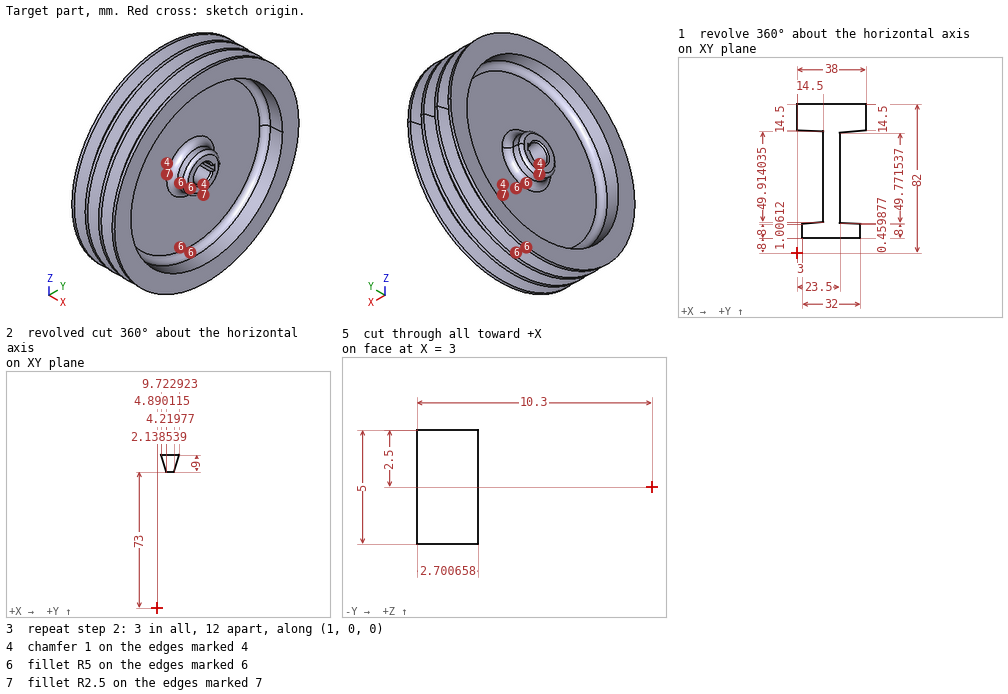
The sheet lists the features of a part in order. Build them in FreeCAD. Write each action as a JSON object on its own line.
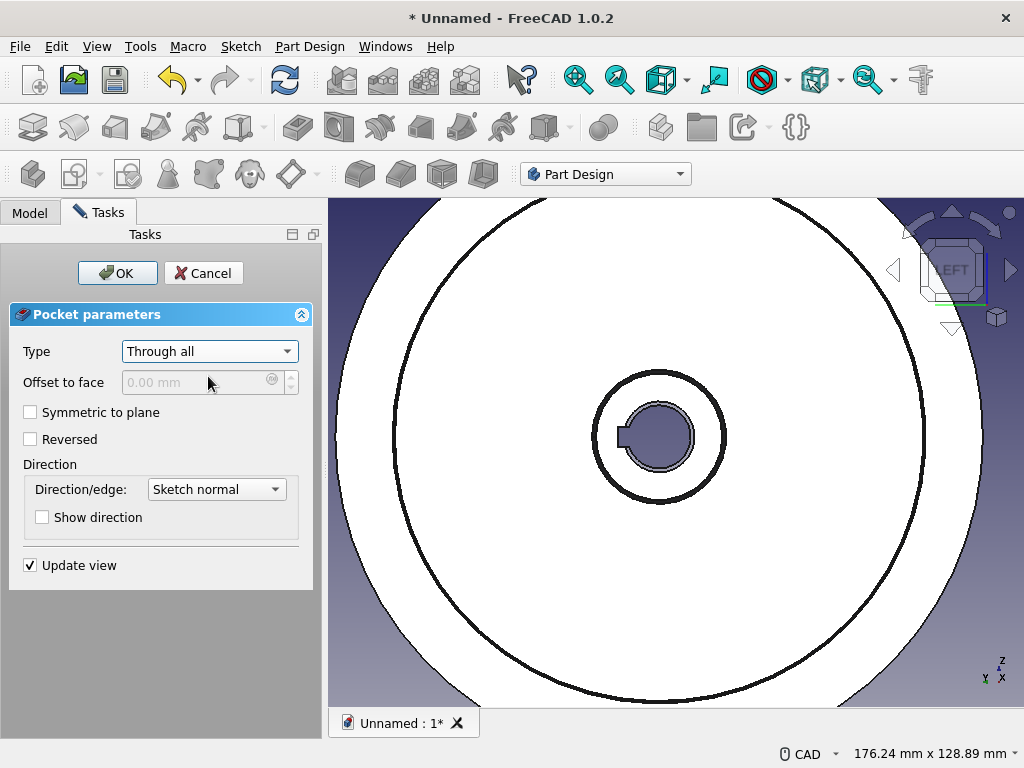
{"action": "left_click", "coordinate": [118, 273]}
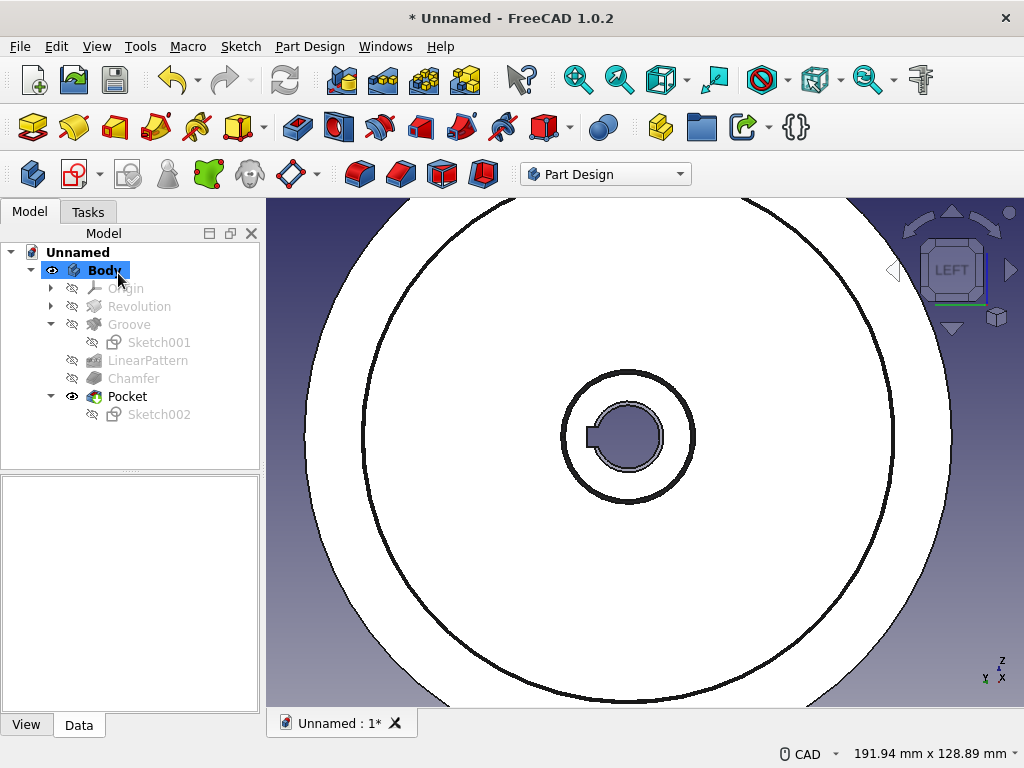
{"action": "left_click", "coordinate": [579, 80]}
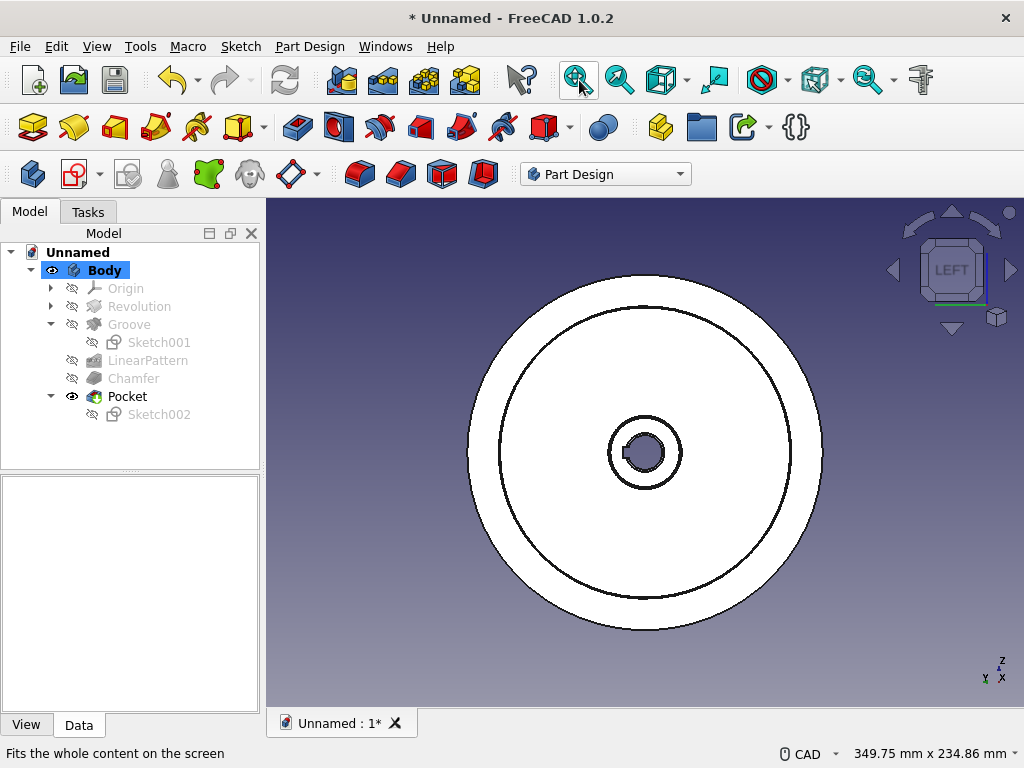
{"action": "key", "text": "0"}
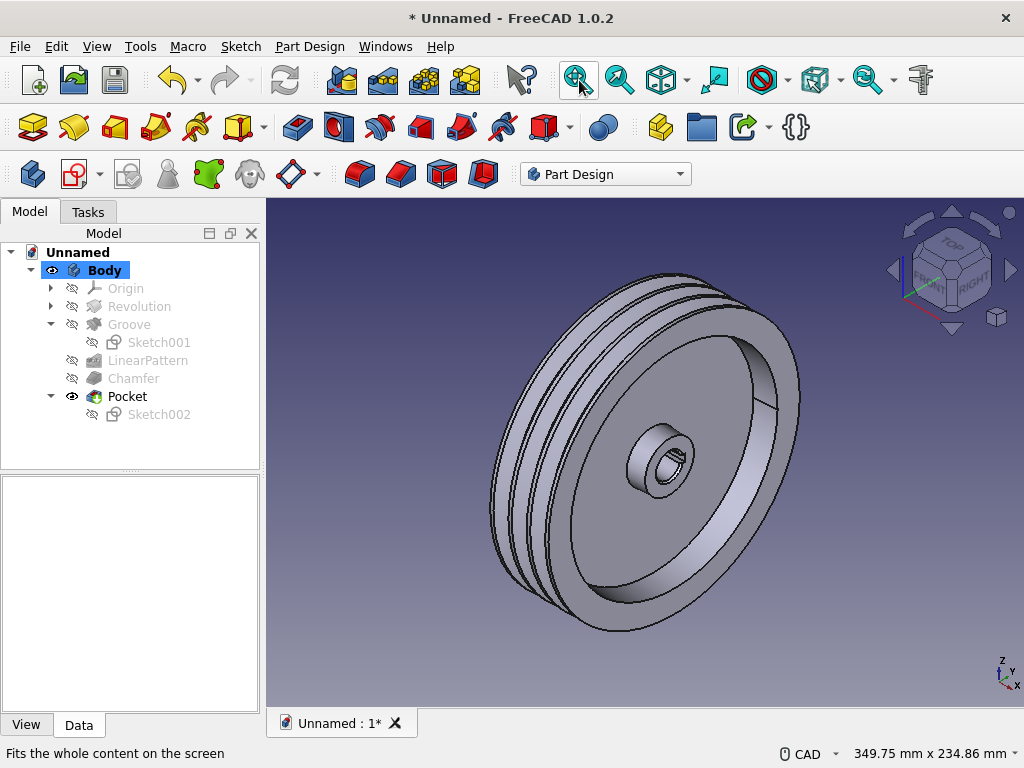
{"action": "key", "text": "2"}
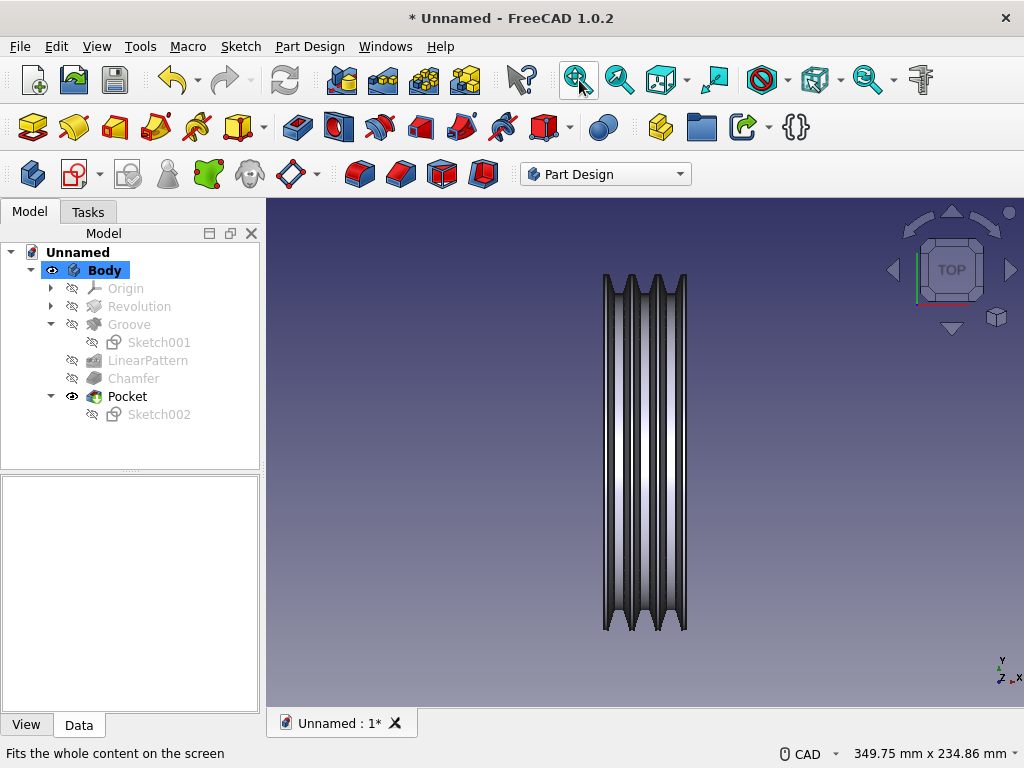
{"action": "key", "text": "1"}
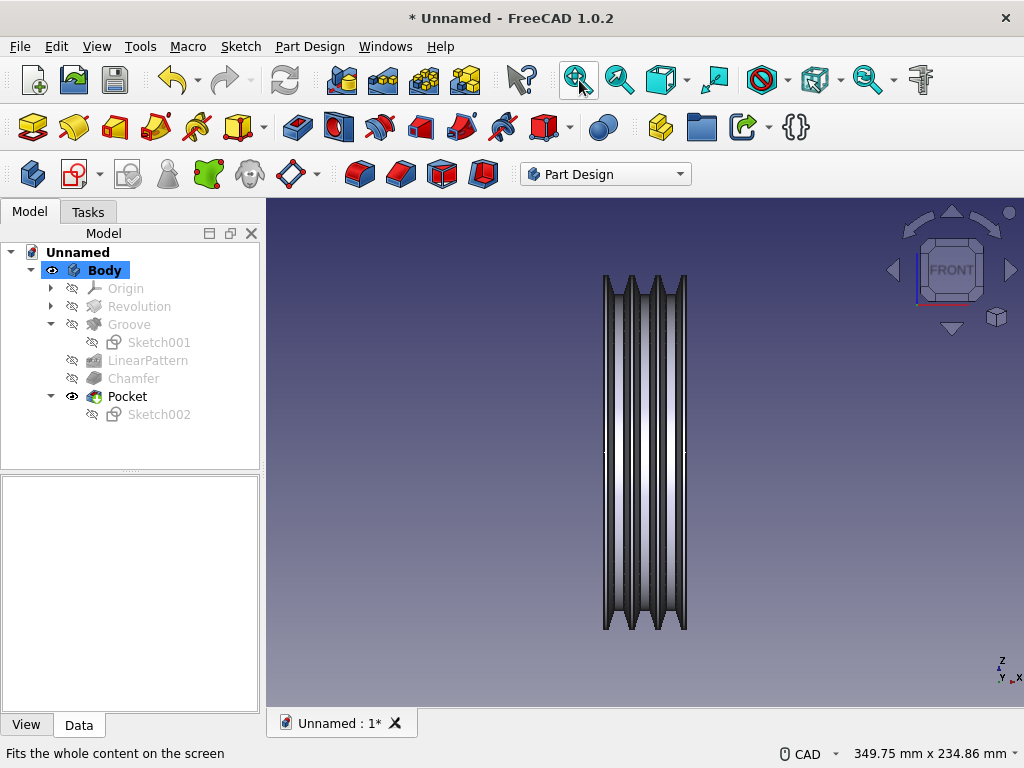
{"action": "key", "text": "3"}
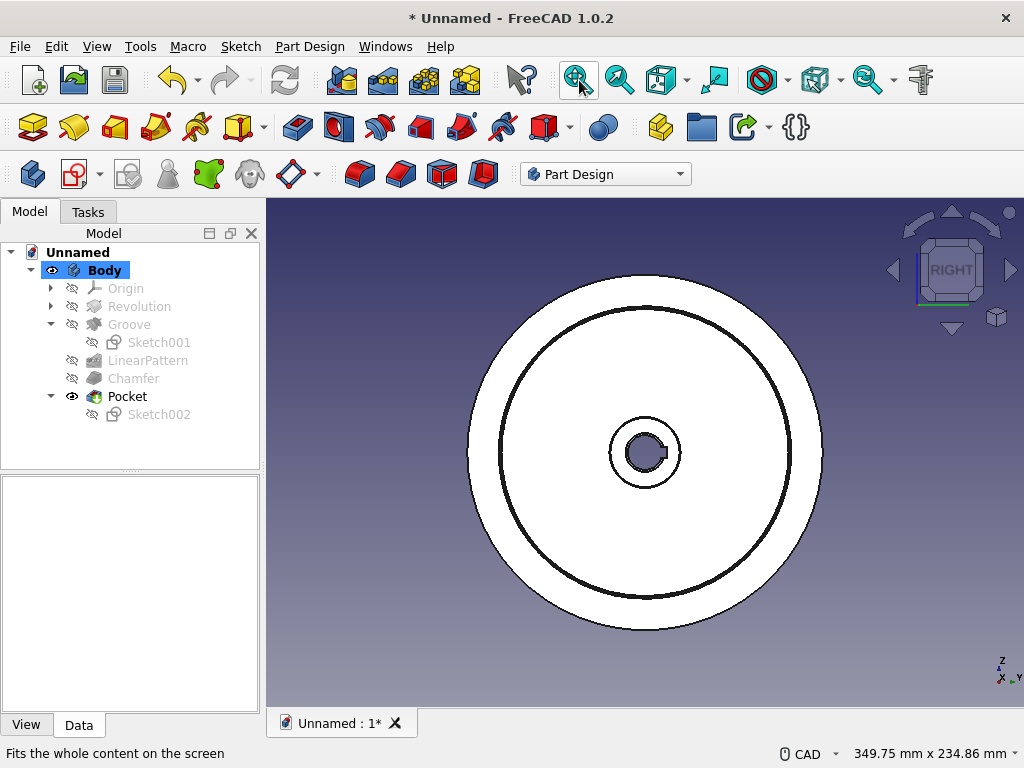
{"action": "key", "text": "5"}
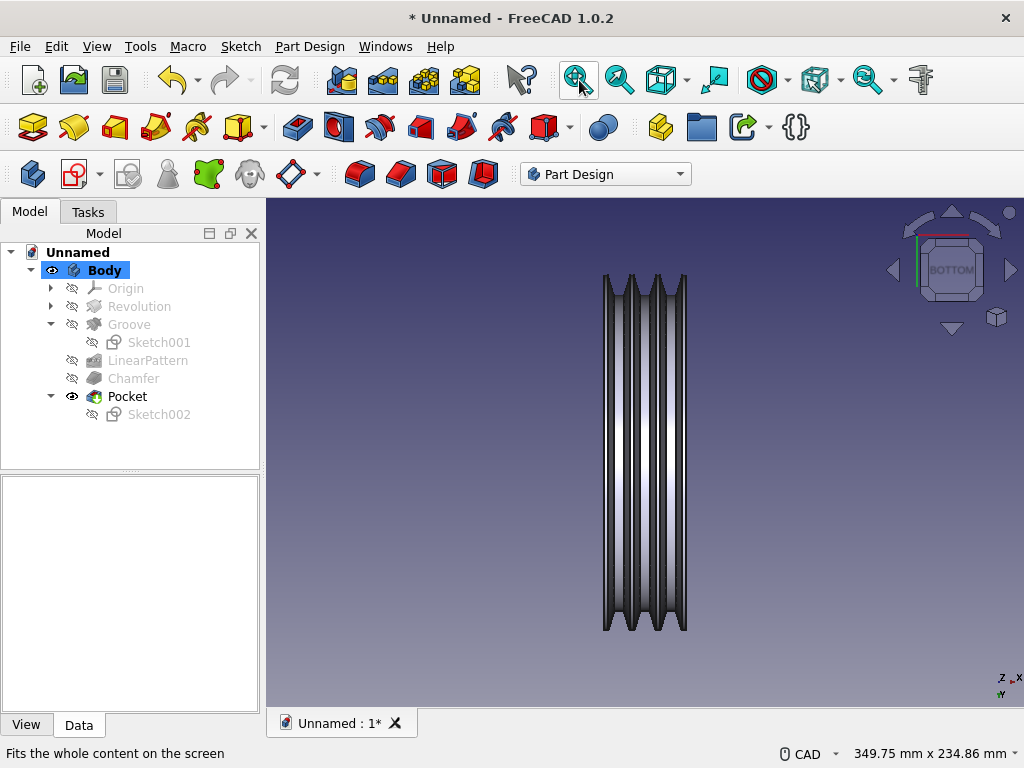
{"action": "key", "text": "4"}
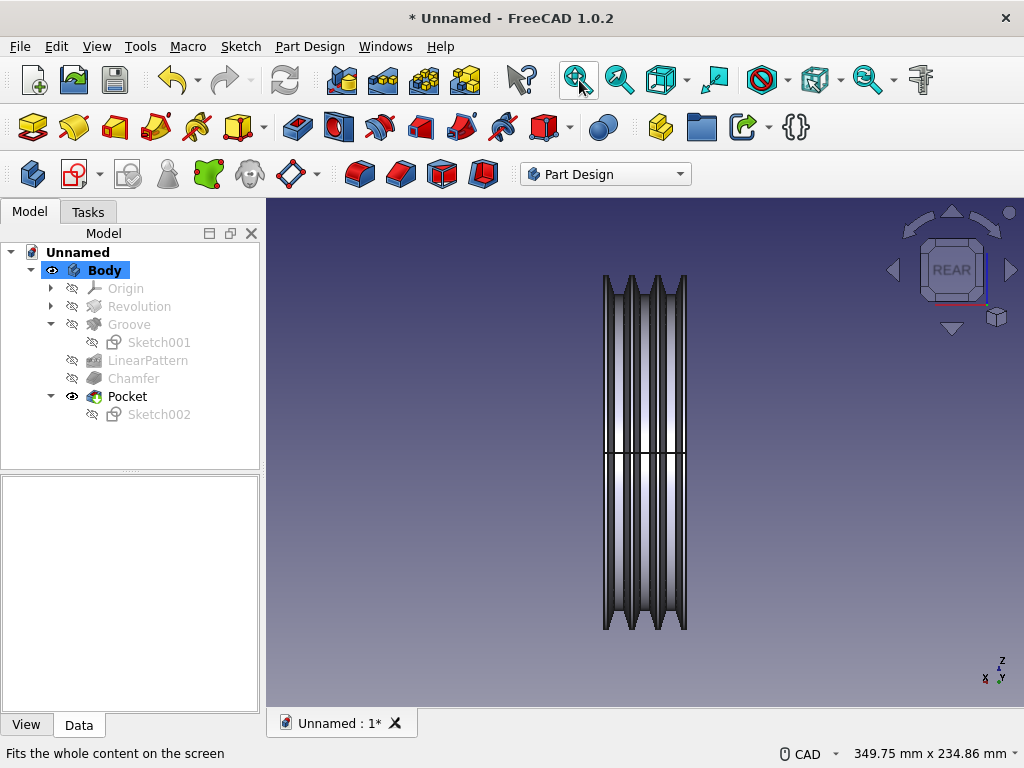
{"action": "key", "text": "6"}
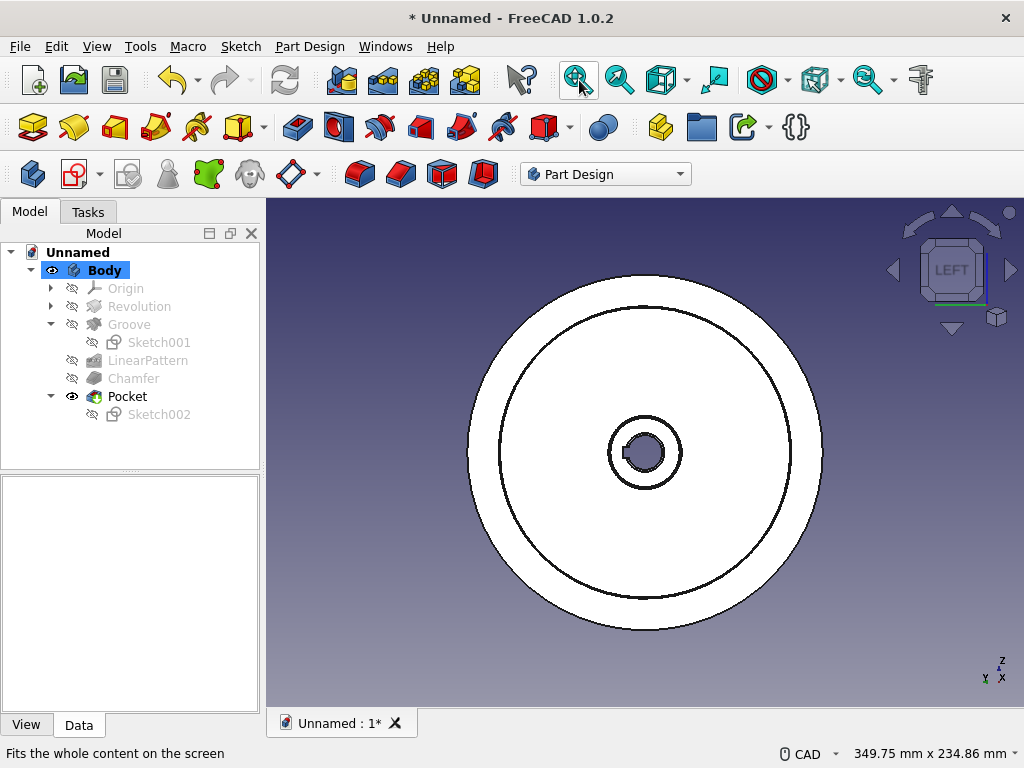
{"action": "key", "text": "v 3"}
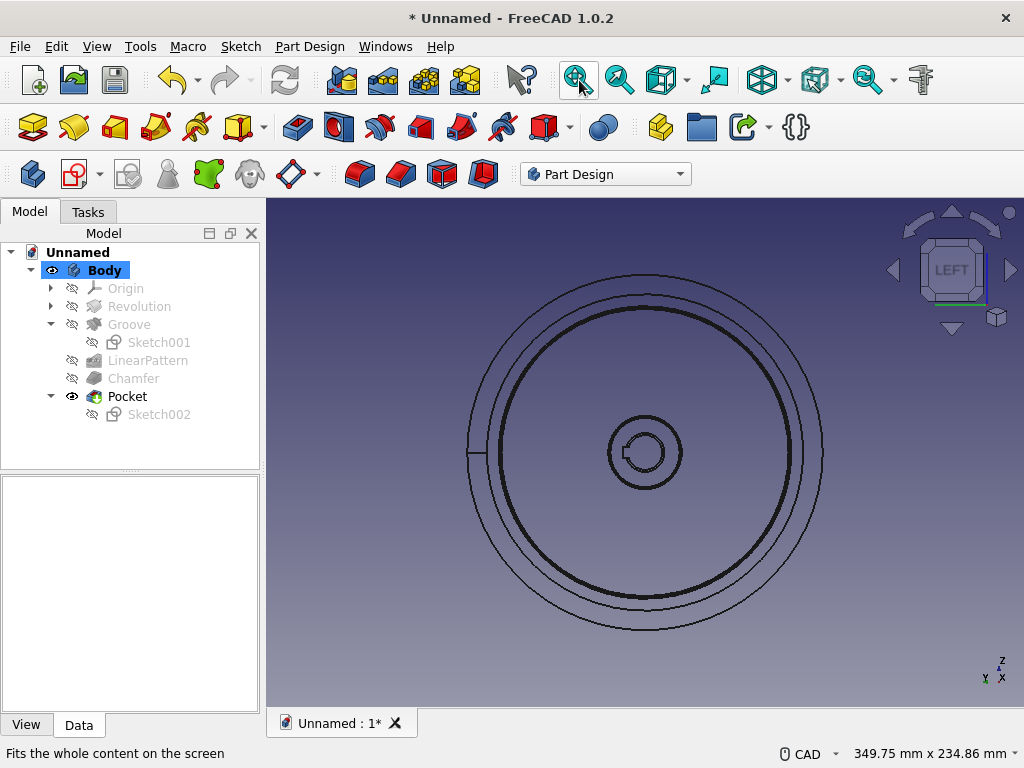
{"action": "key", "text": "0"}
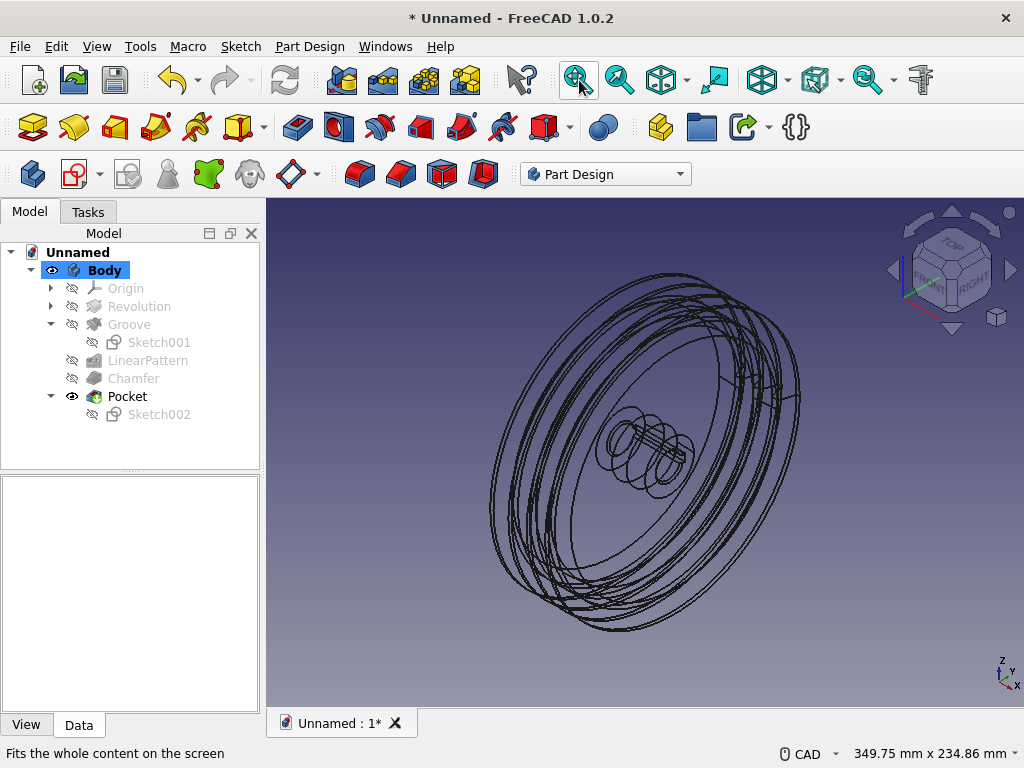
{"action": "left_click", "coordinate": [606, 578]}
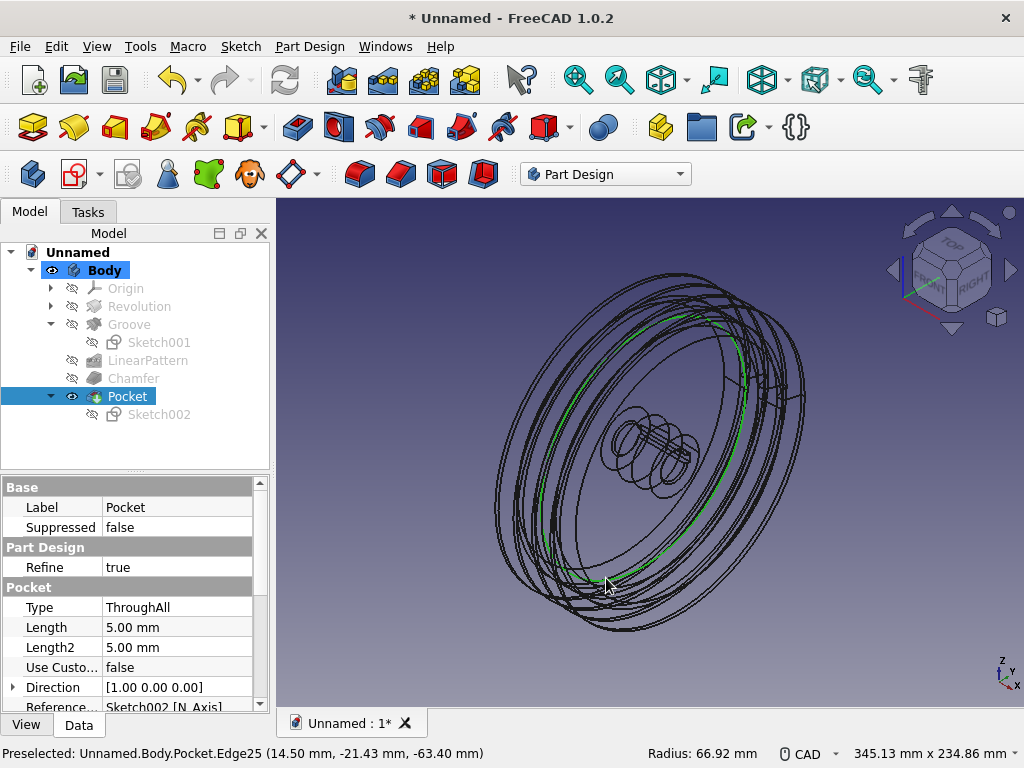
{"action": "left_click", "coordinate": [617, 463], "text": "ctrl"}